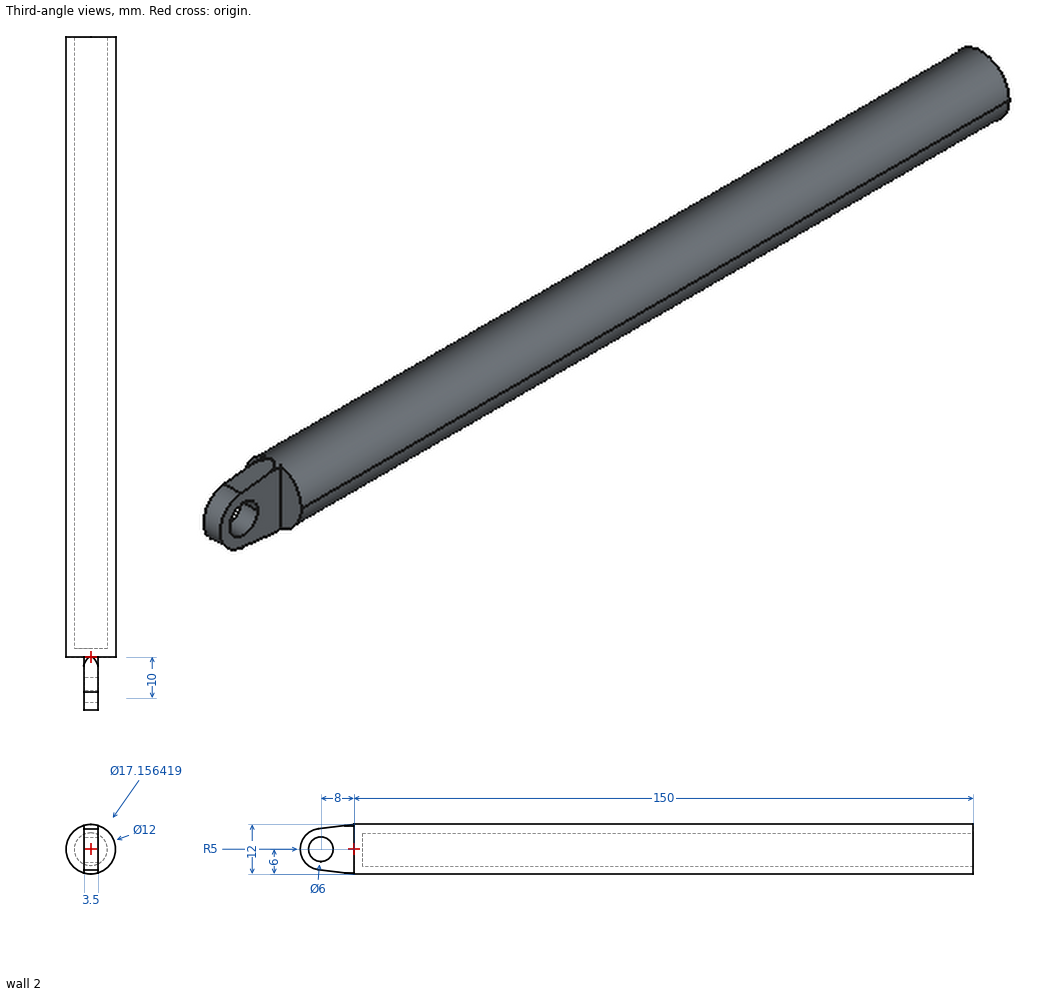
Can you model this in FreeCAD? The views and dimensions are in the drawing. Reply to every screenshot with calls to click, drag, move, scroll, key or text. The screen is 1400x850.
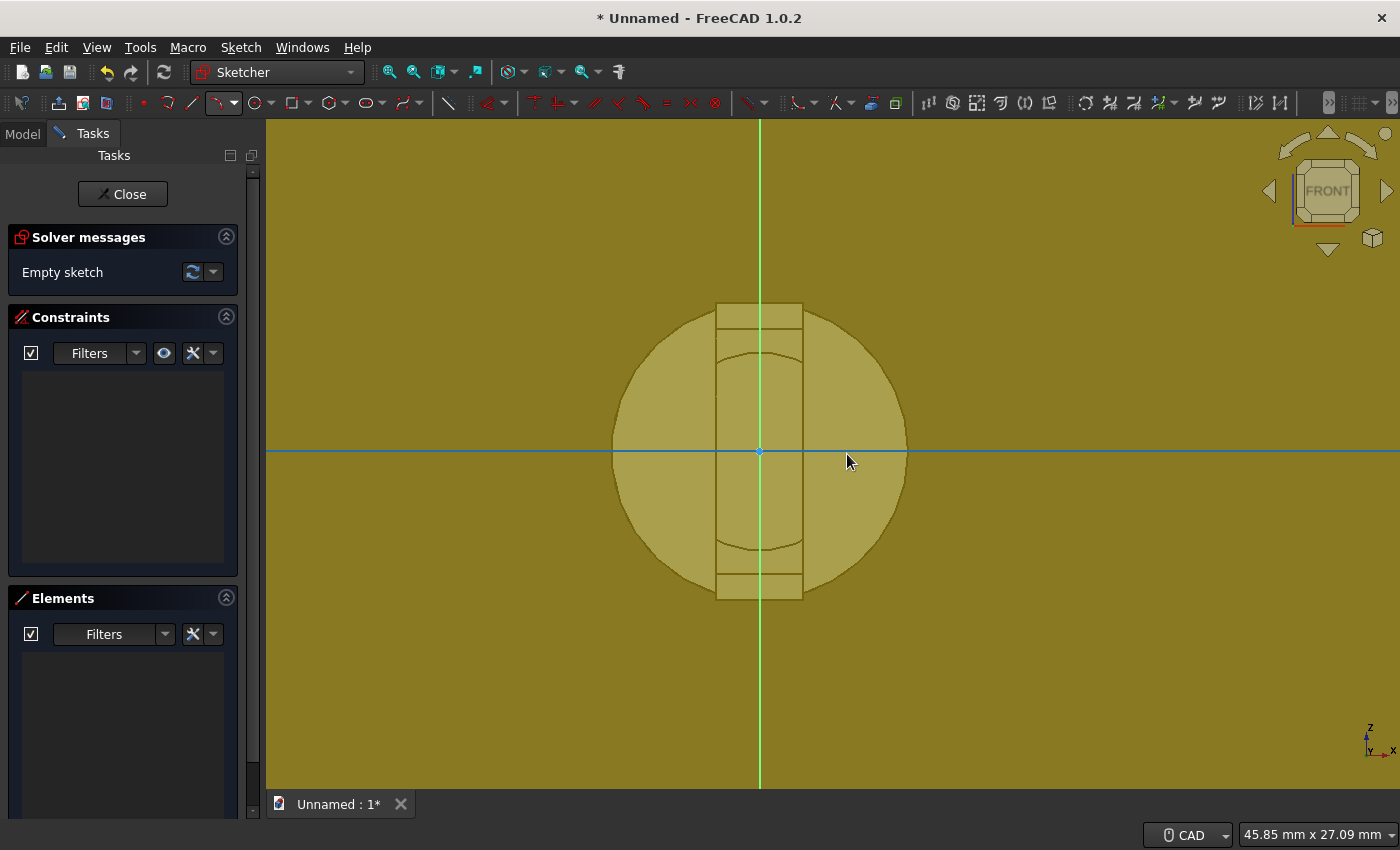
click(256, 104)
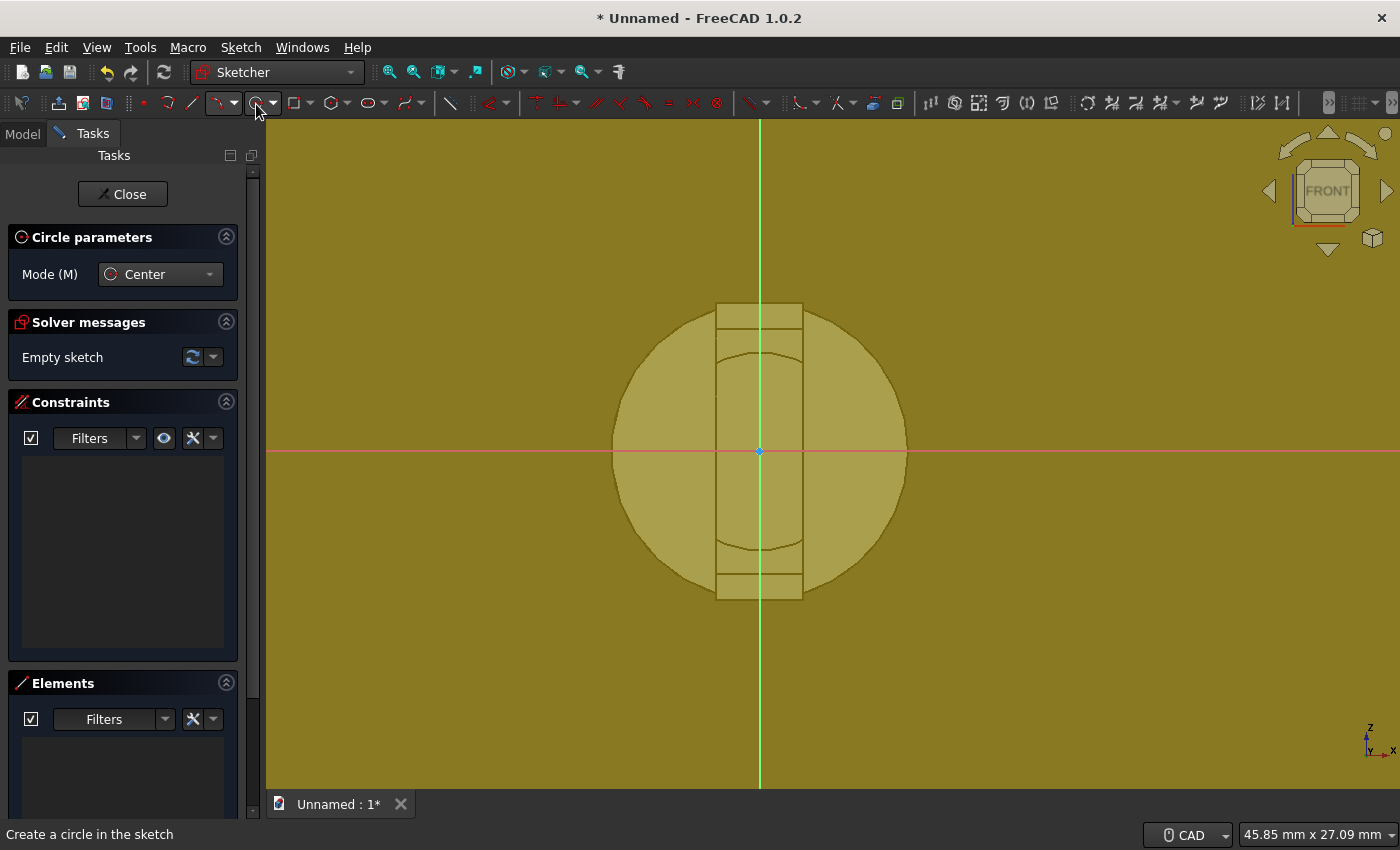
click(760, 451)
click(910, 301)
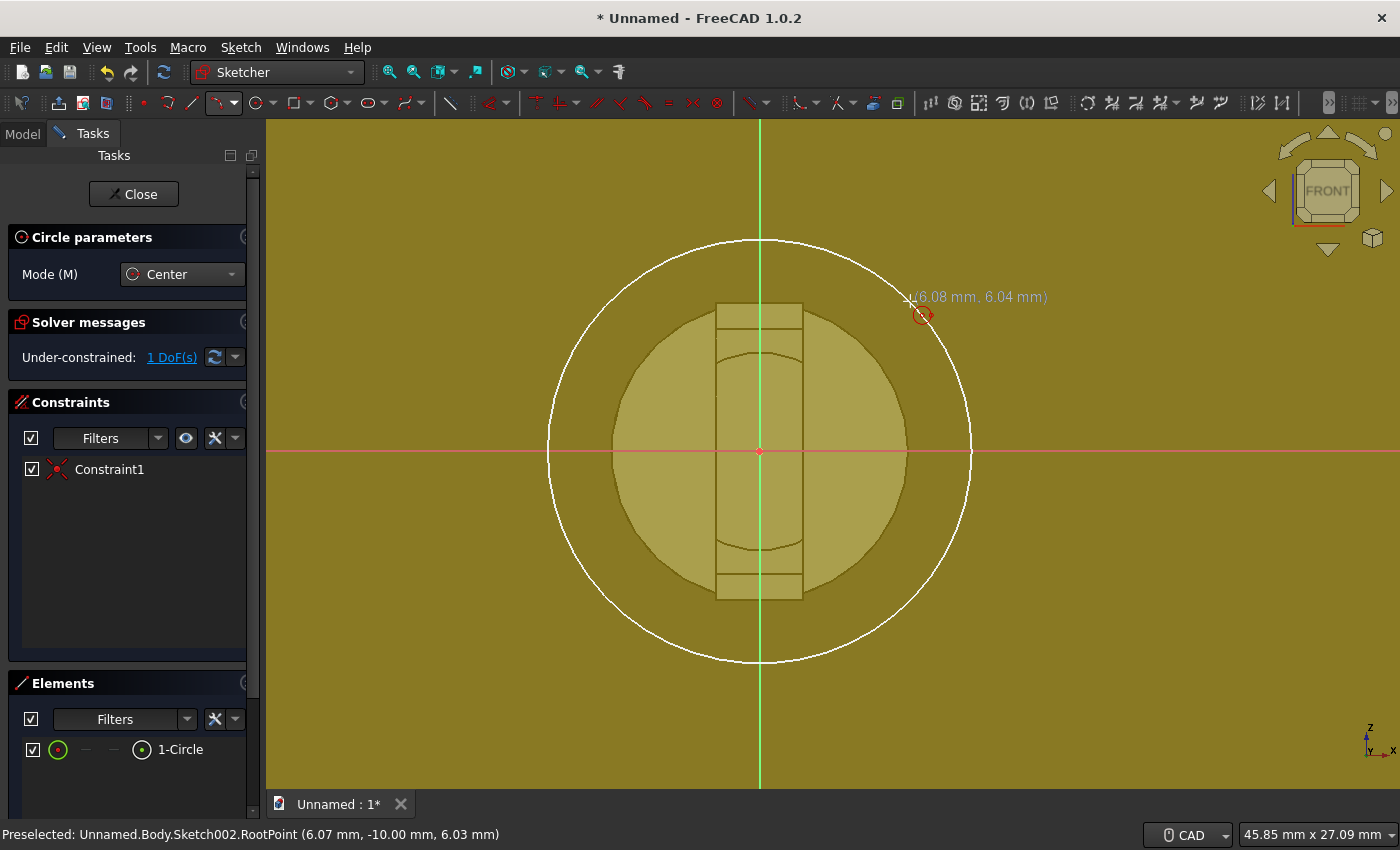
click(760, 451)
click(865, 347)
key(Escape)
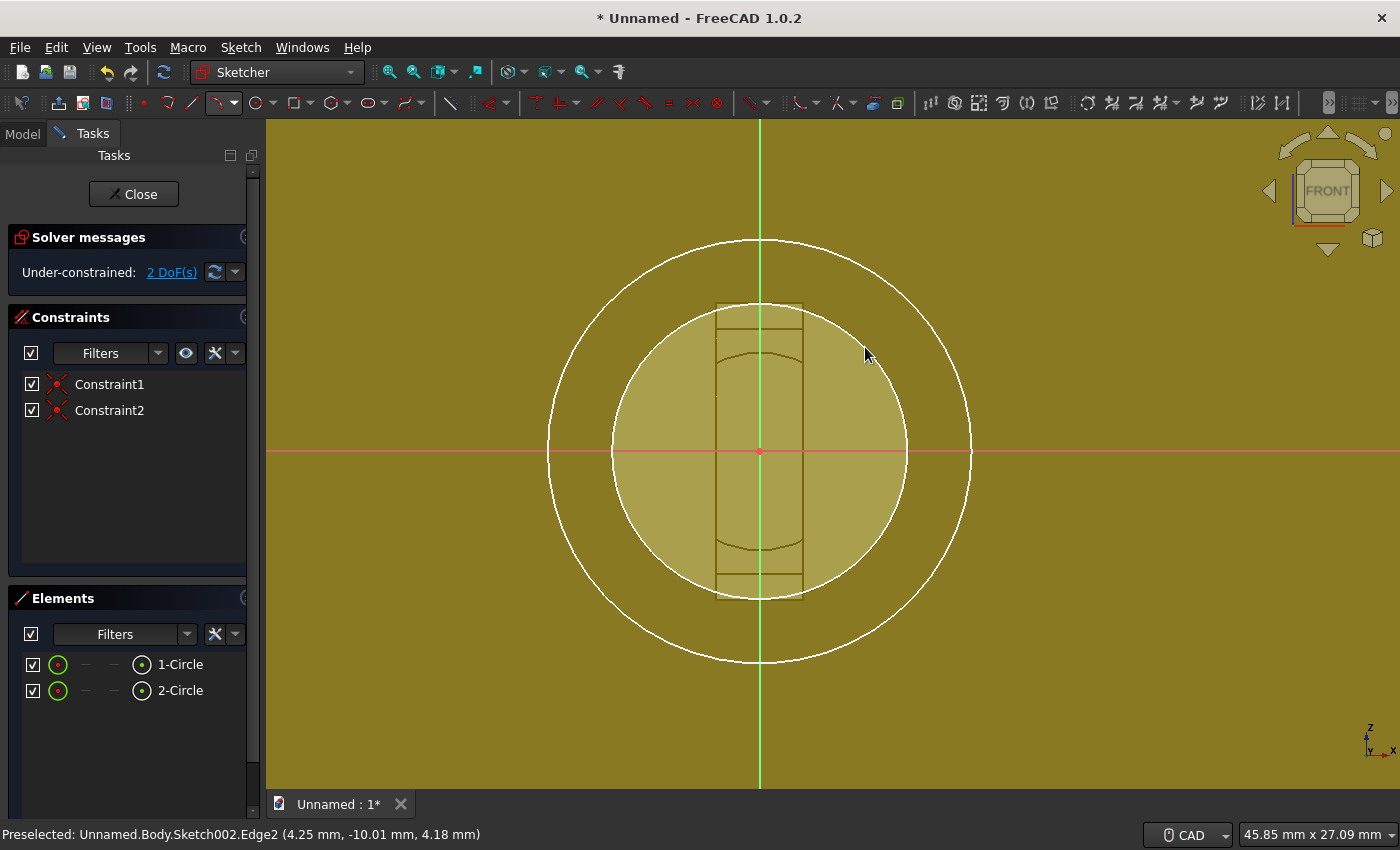
click(490, 104)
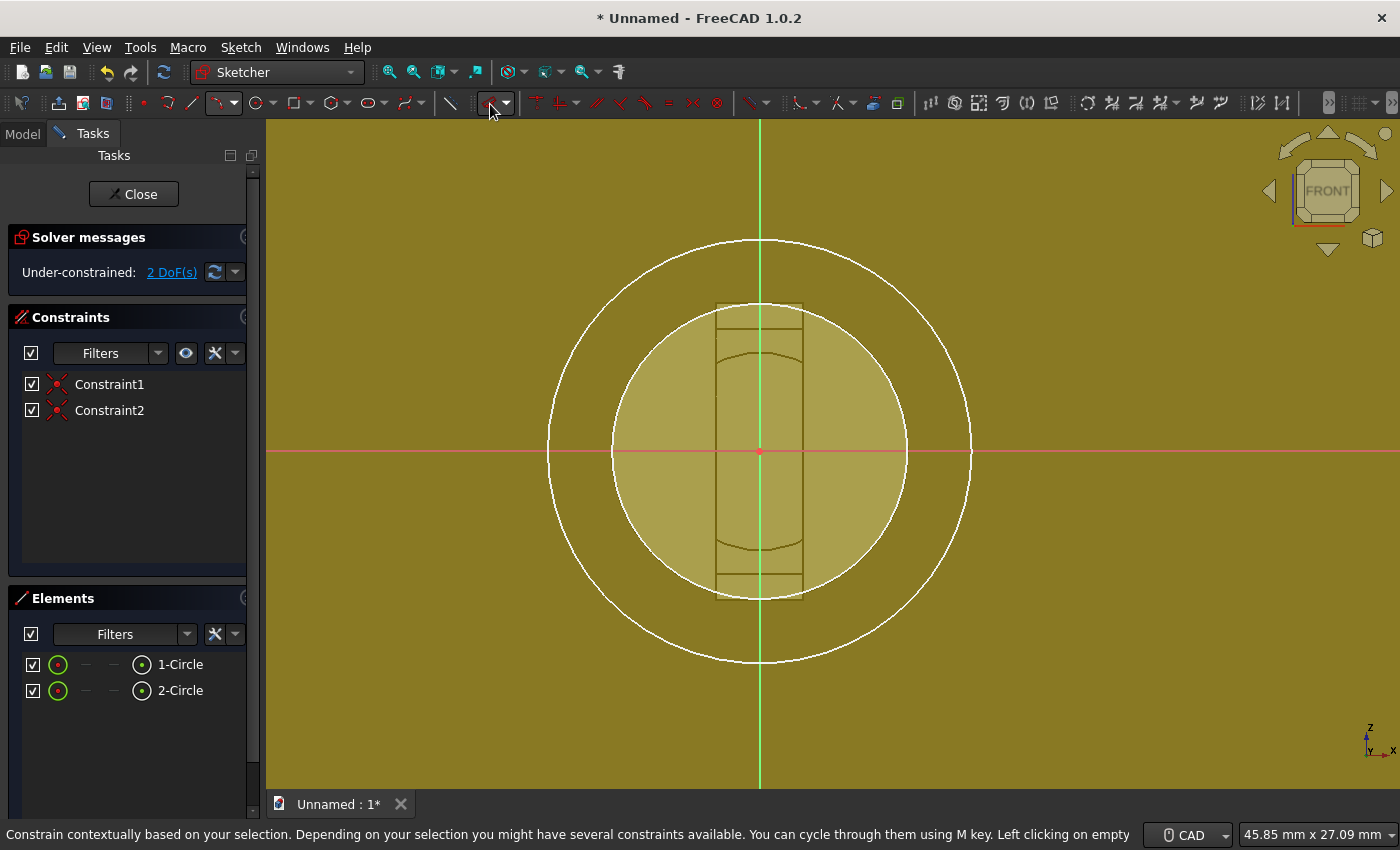
click(909, 301)
click(932, 278)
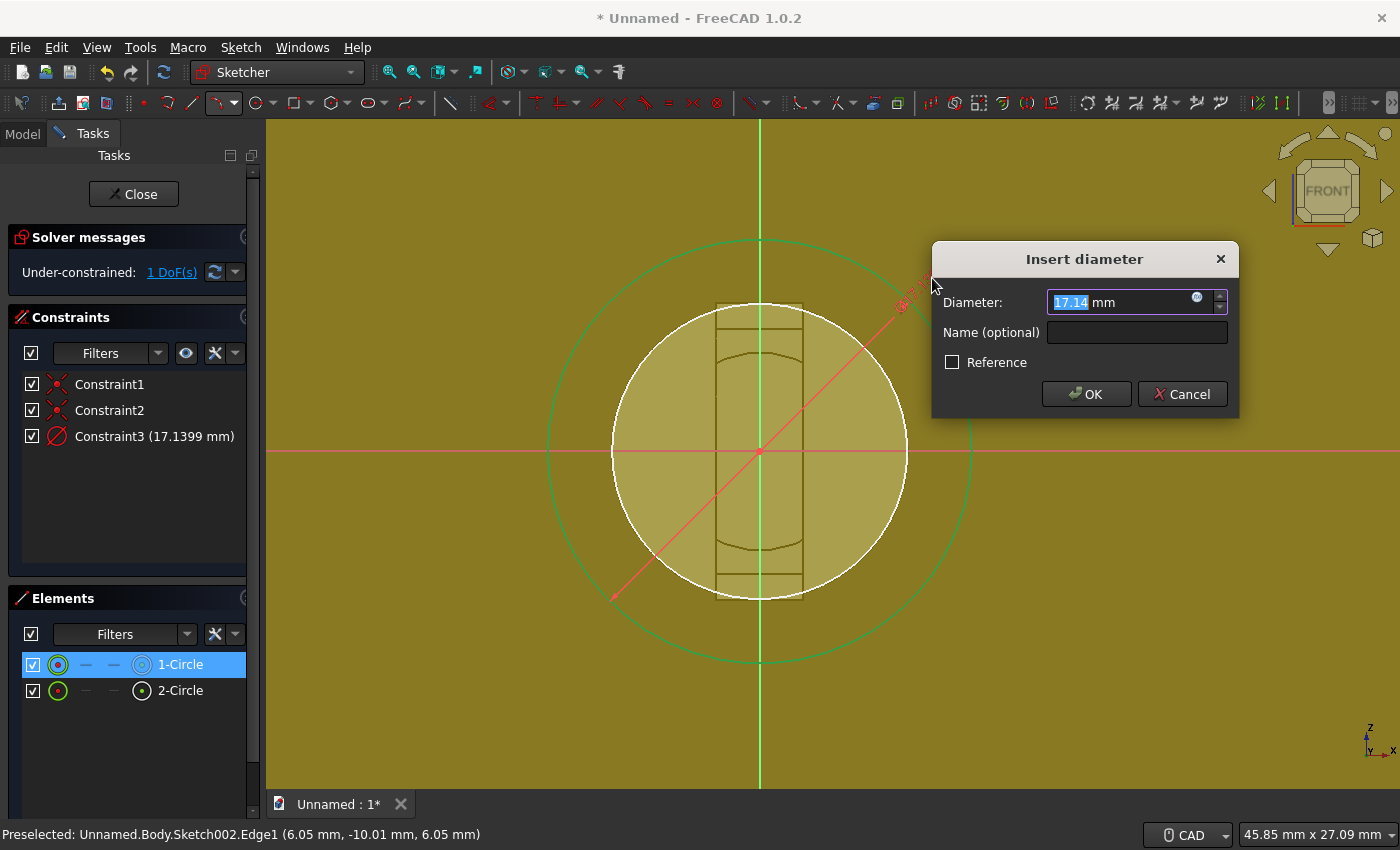
text(17.156419)
key(Return)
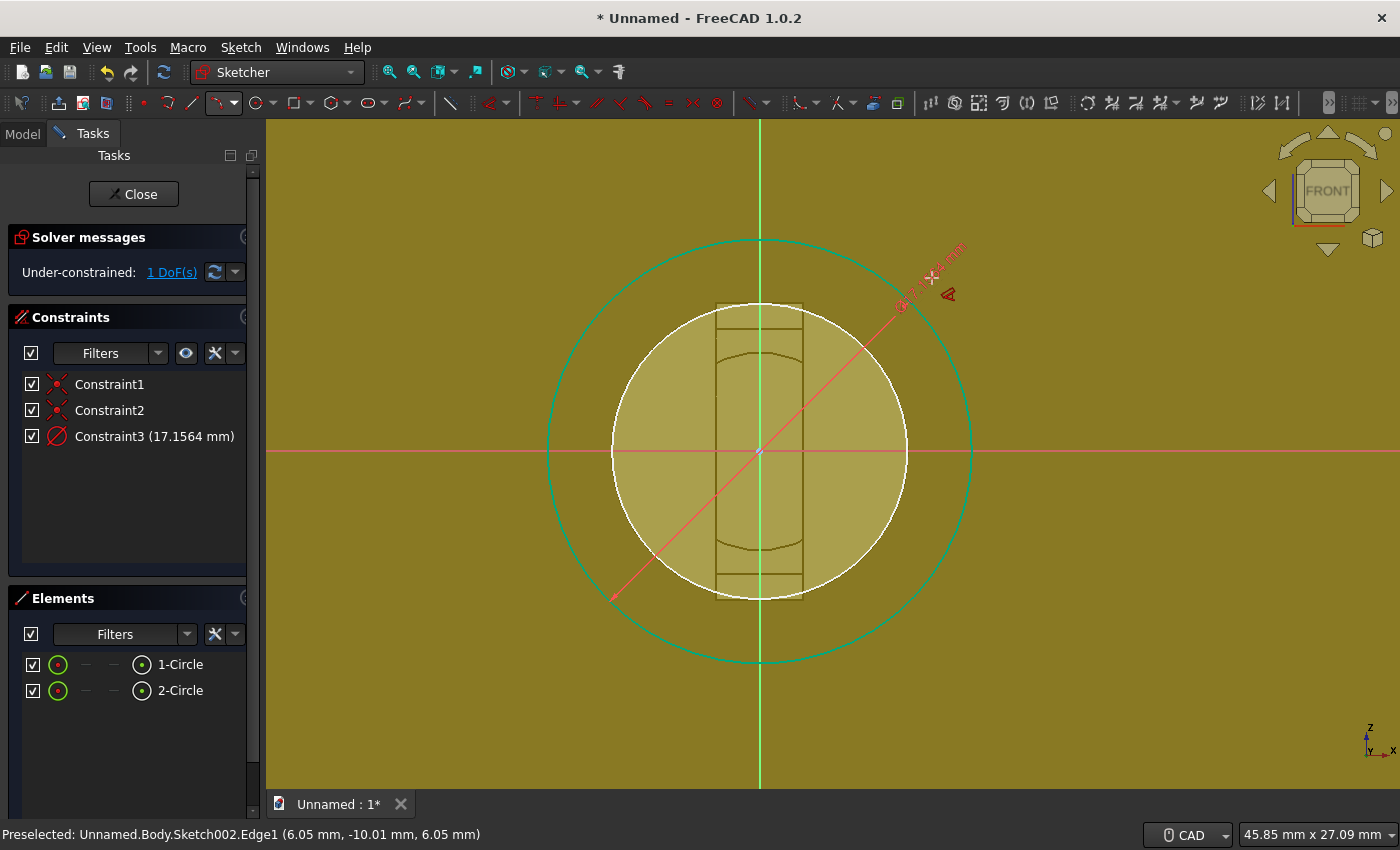
click(864, 347)
click(887, 324)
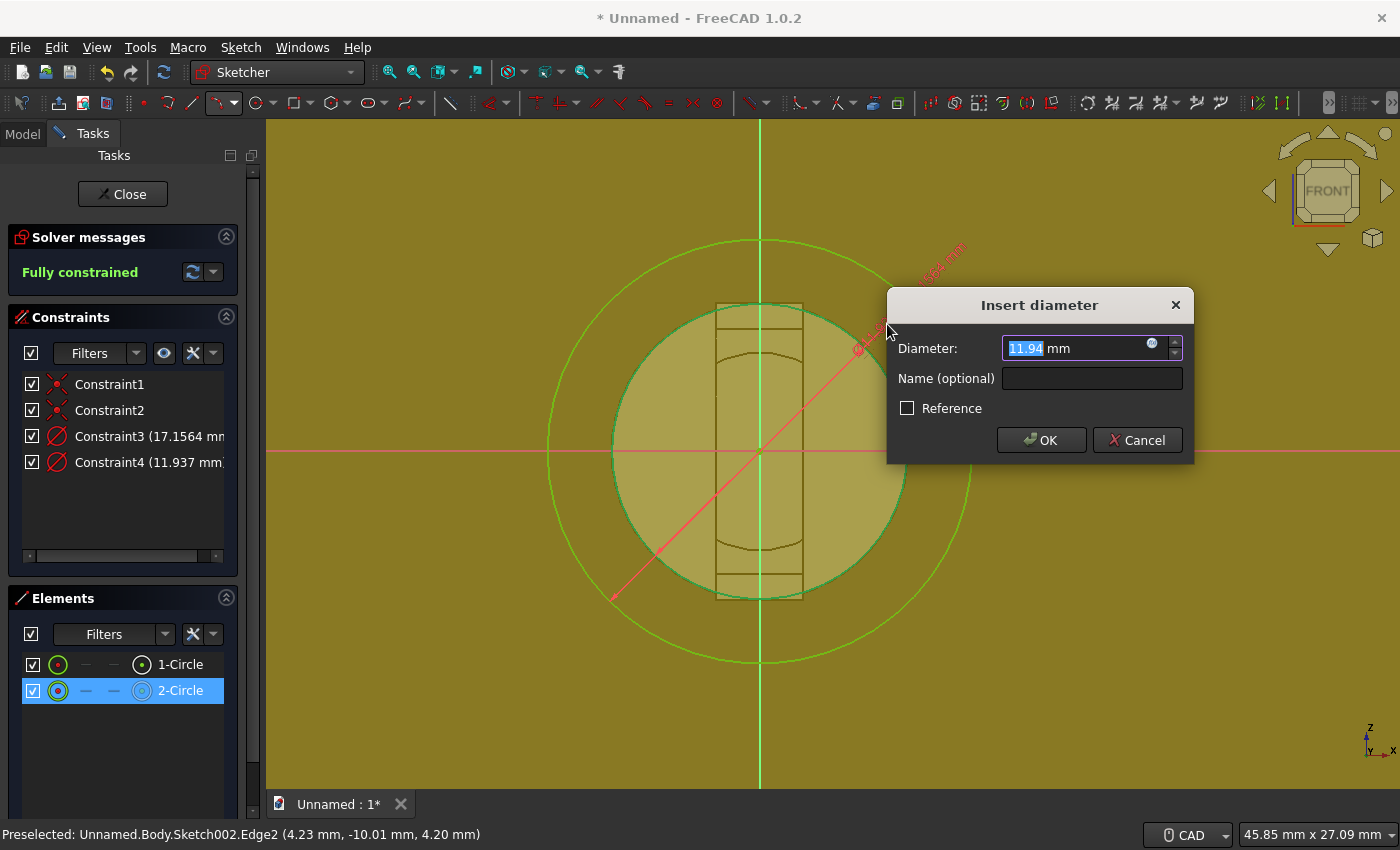
text(12)
key(Return)
key(Escape)